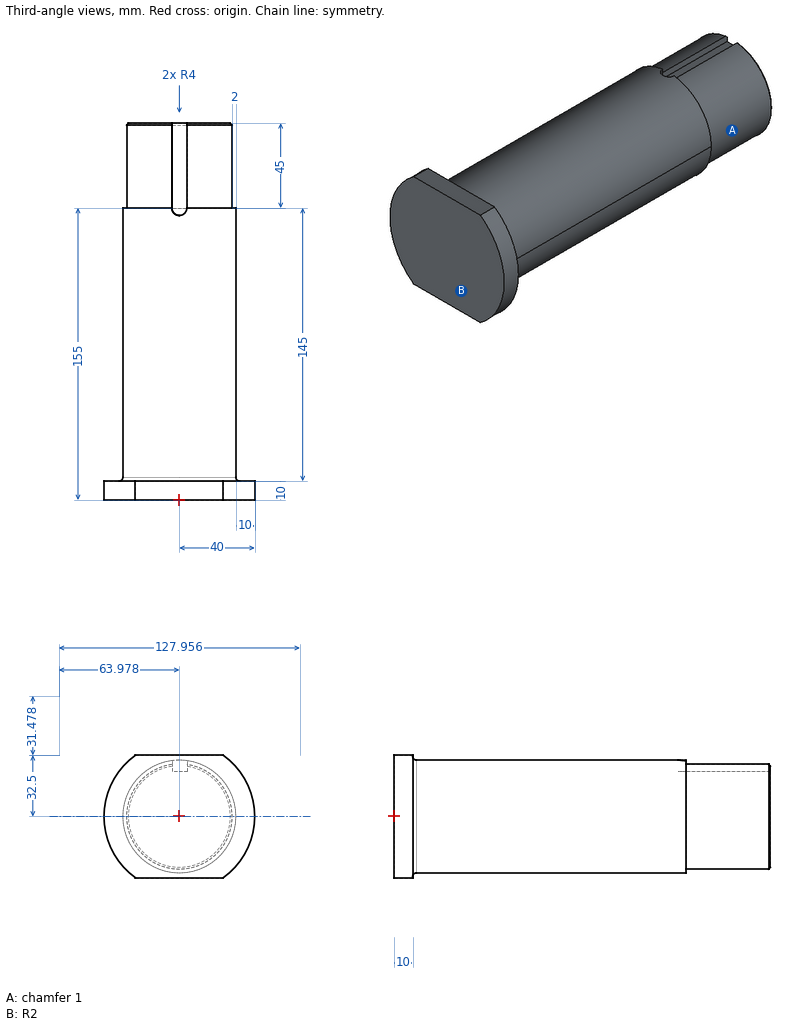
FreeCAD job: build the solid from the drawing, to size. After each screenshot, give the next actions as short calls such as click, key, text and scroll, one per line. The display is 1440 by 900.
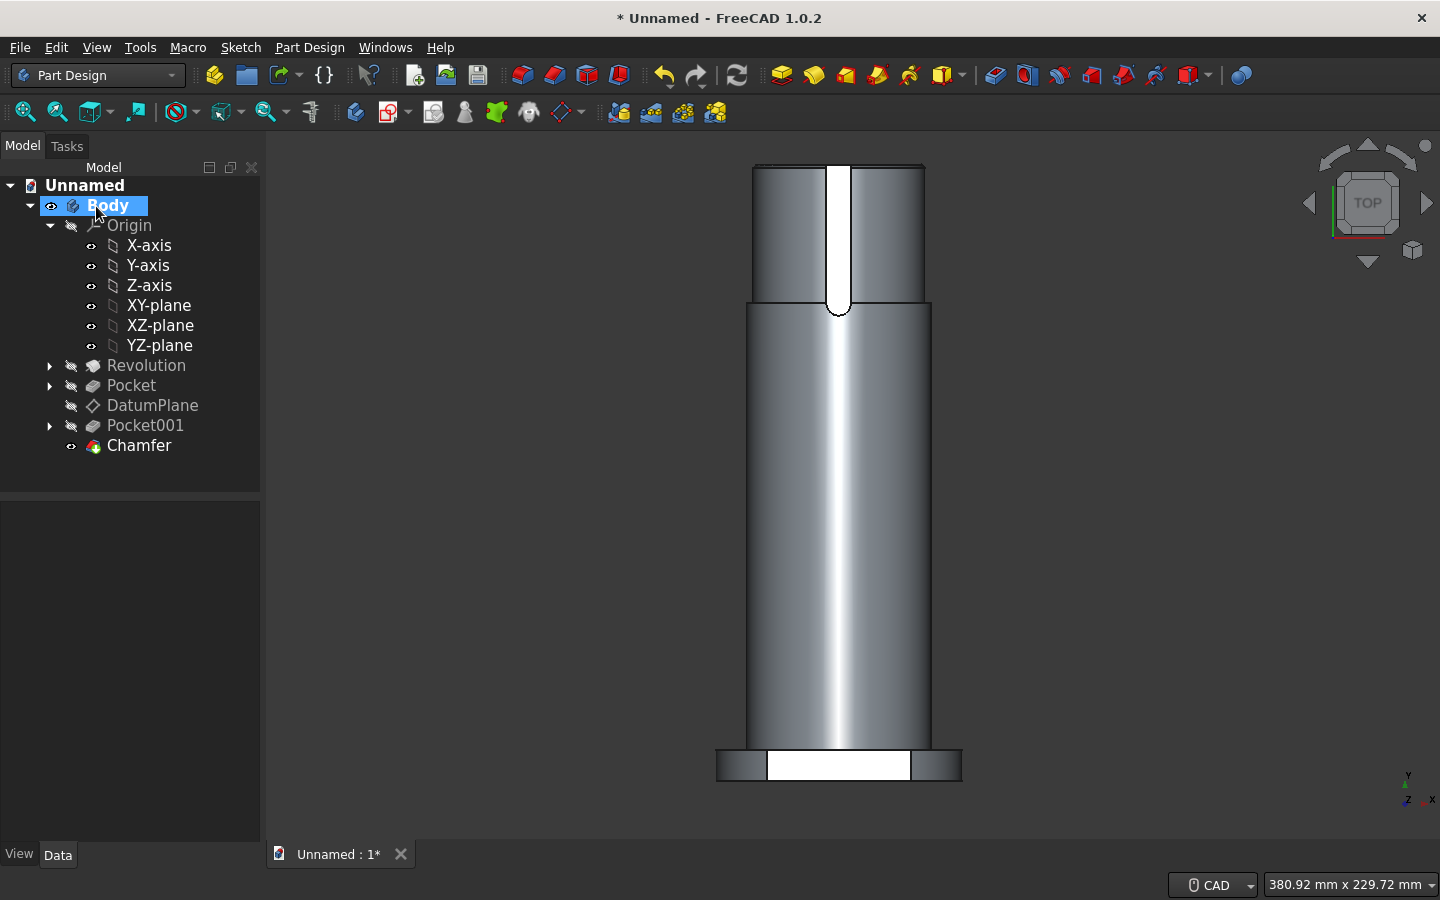
key(0)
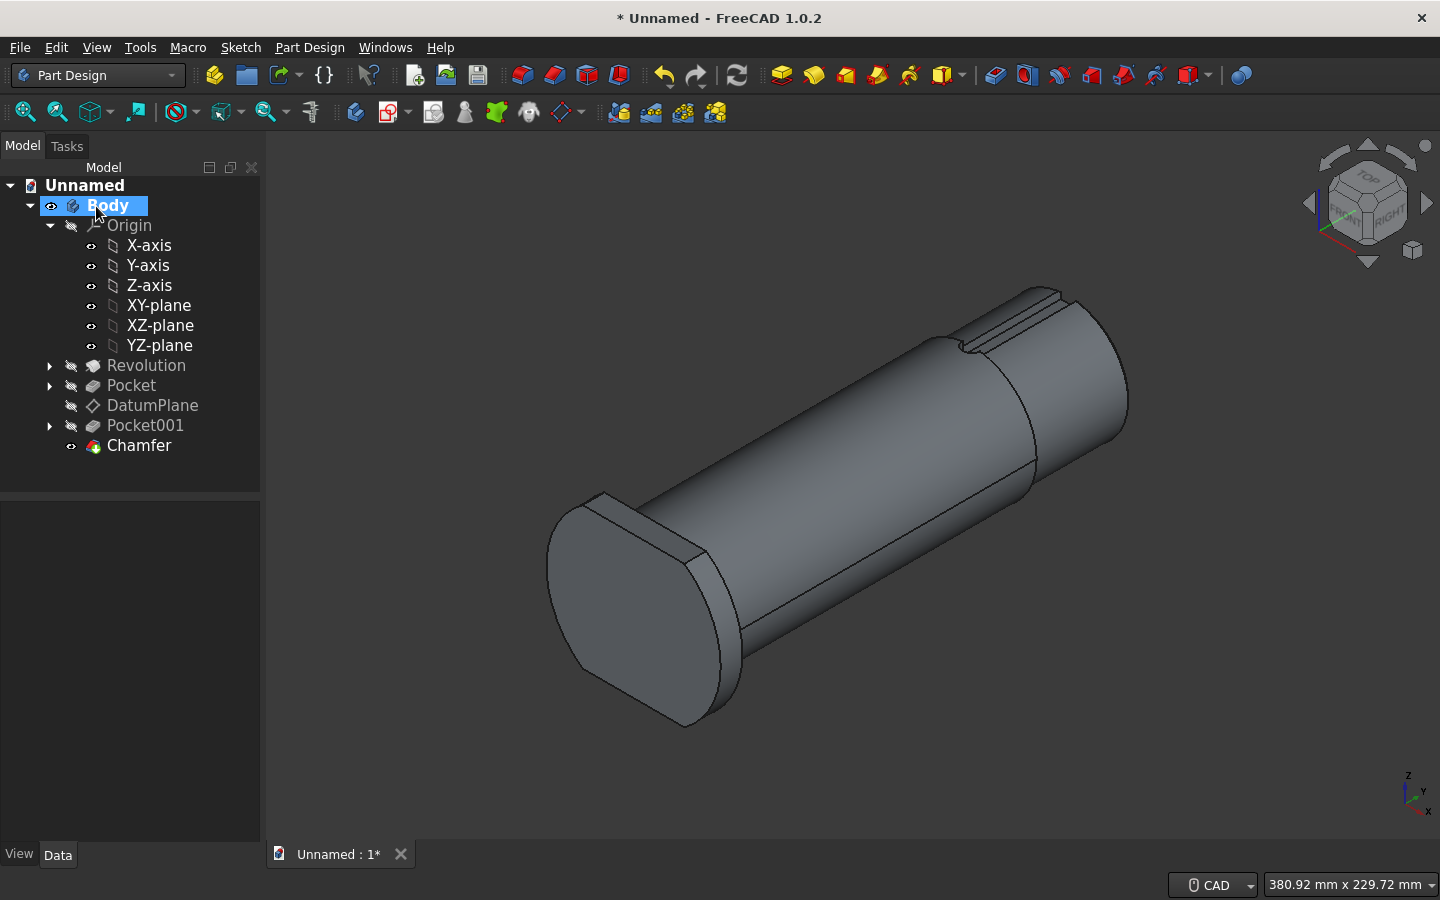
key(2)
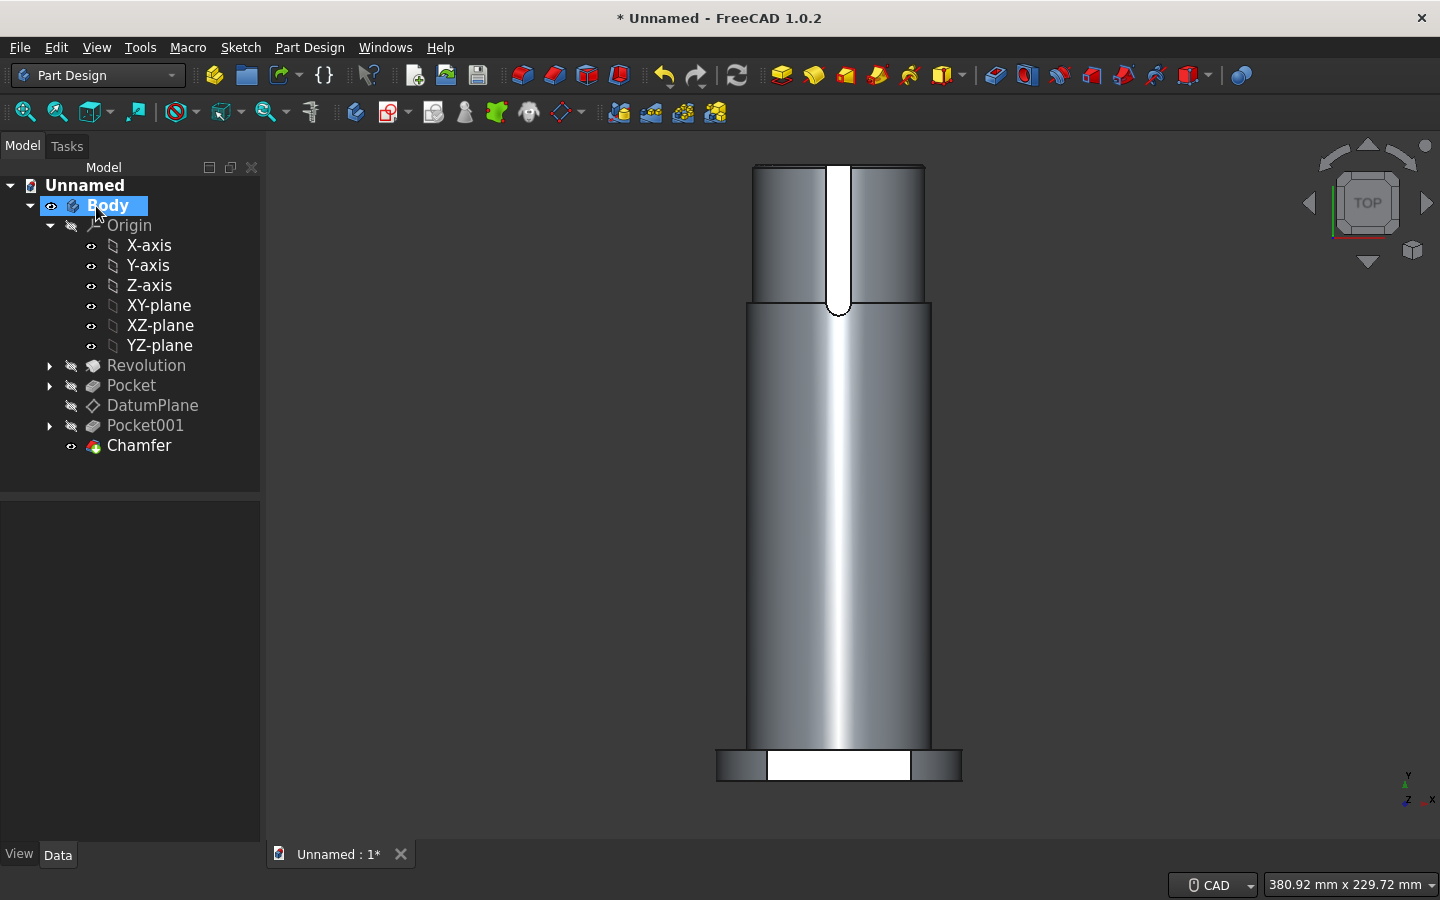
key(1)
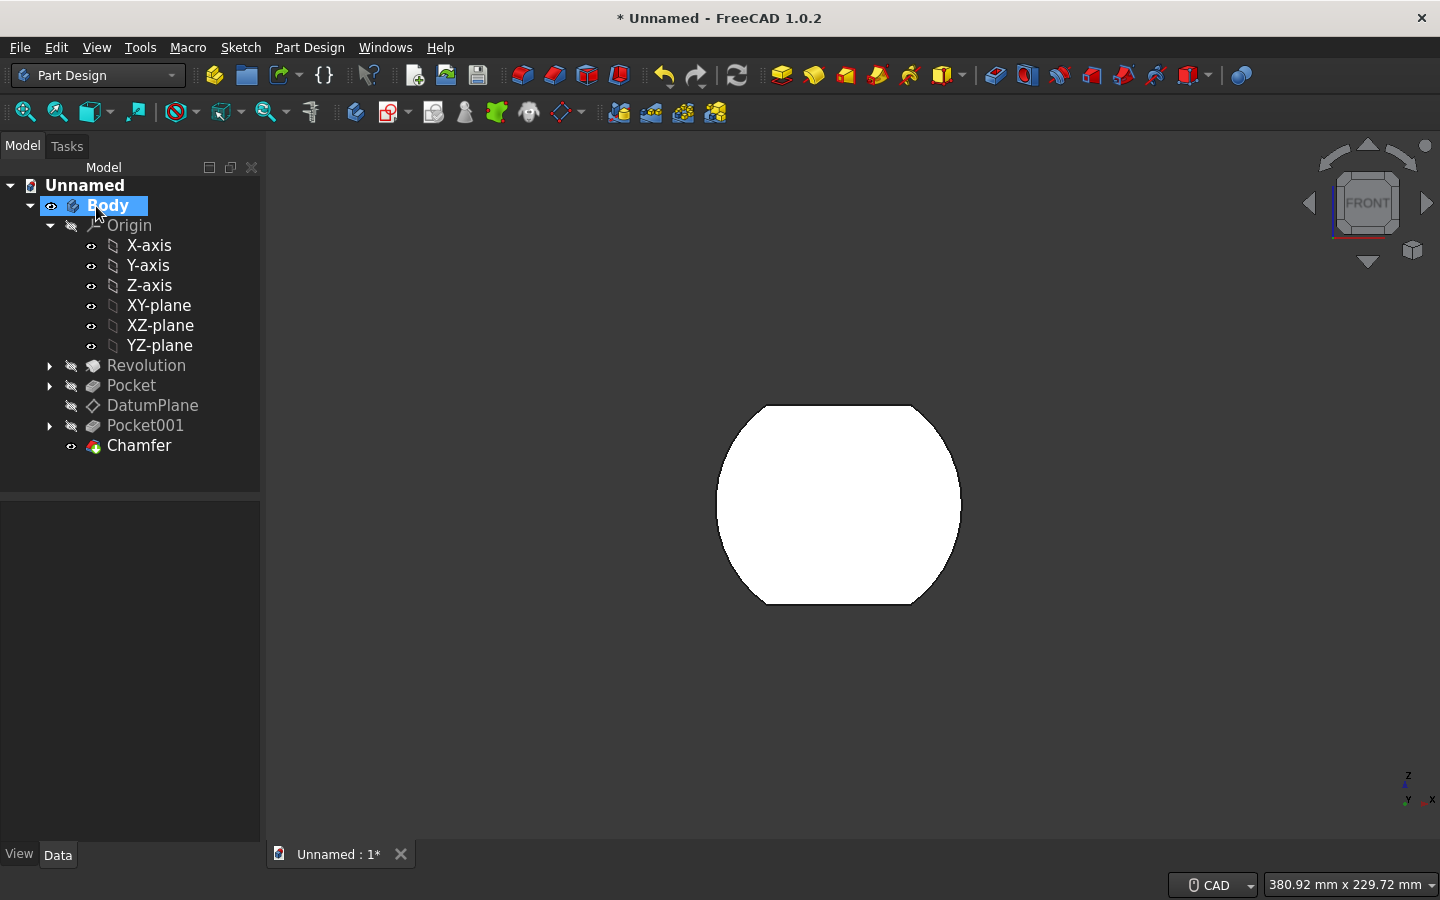
click(26, 112)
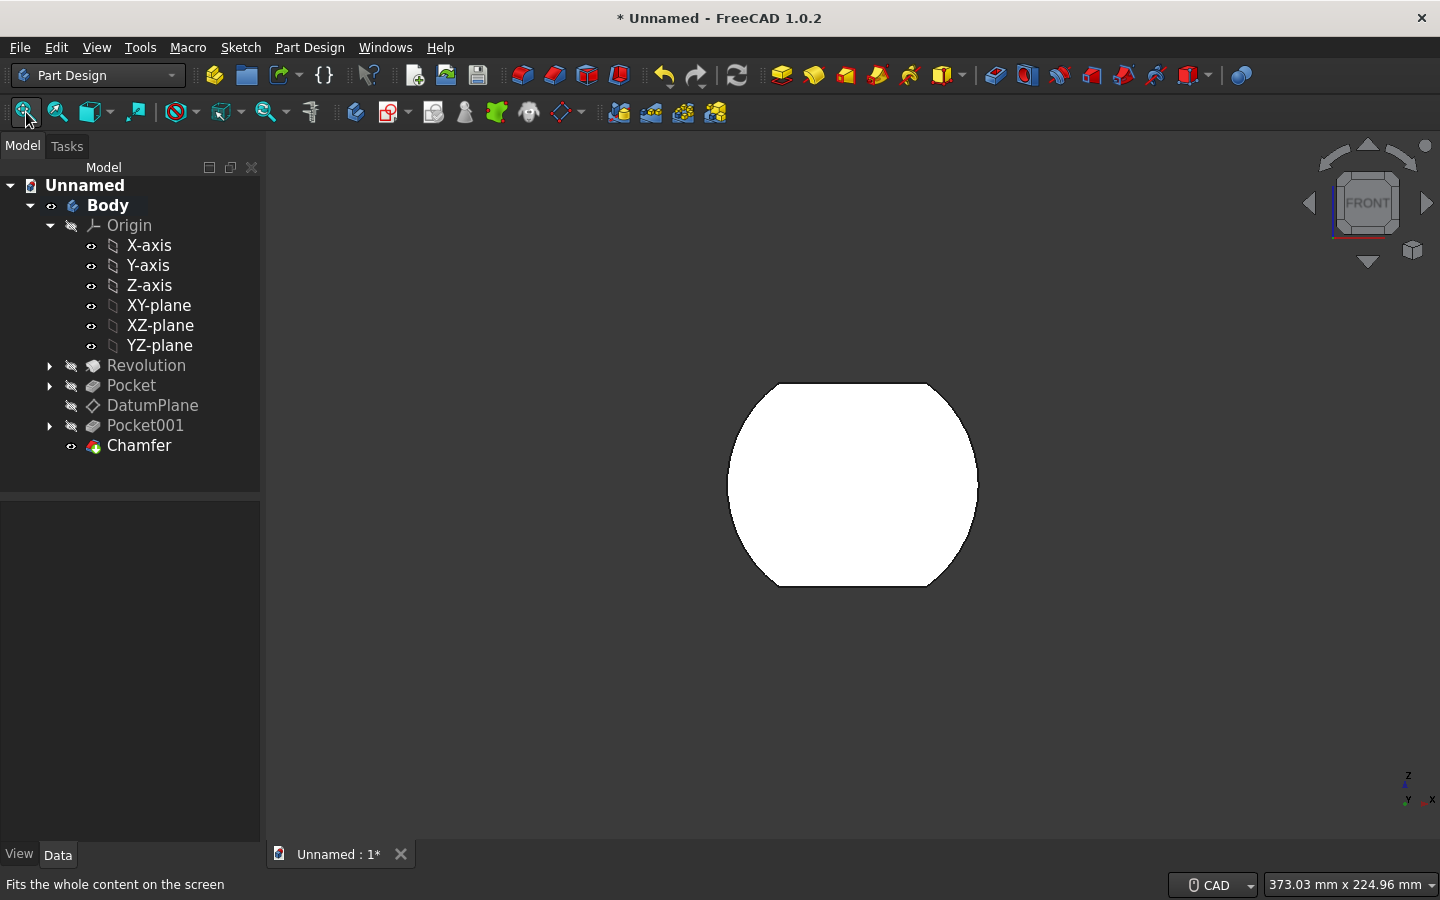
key(3)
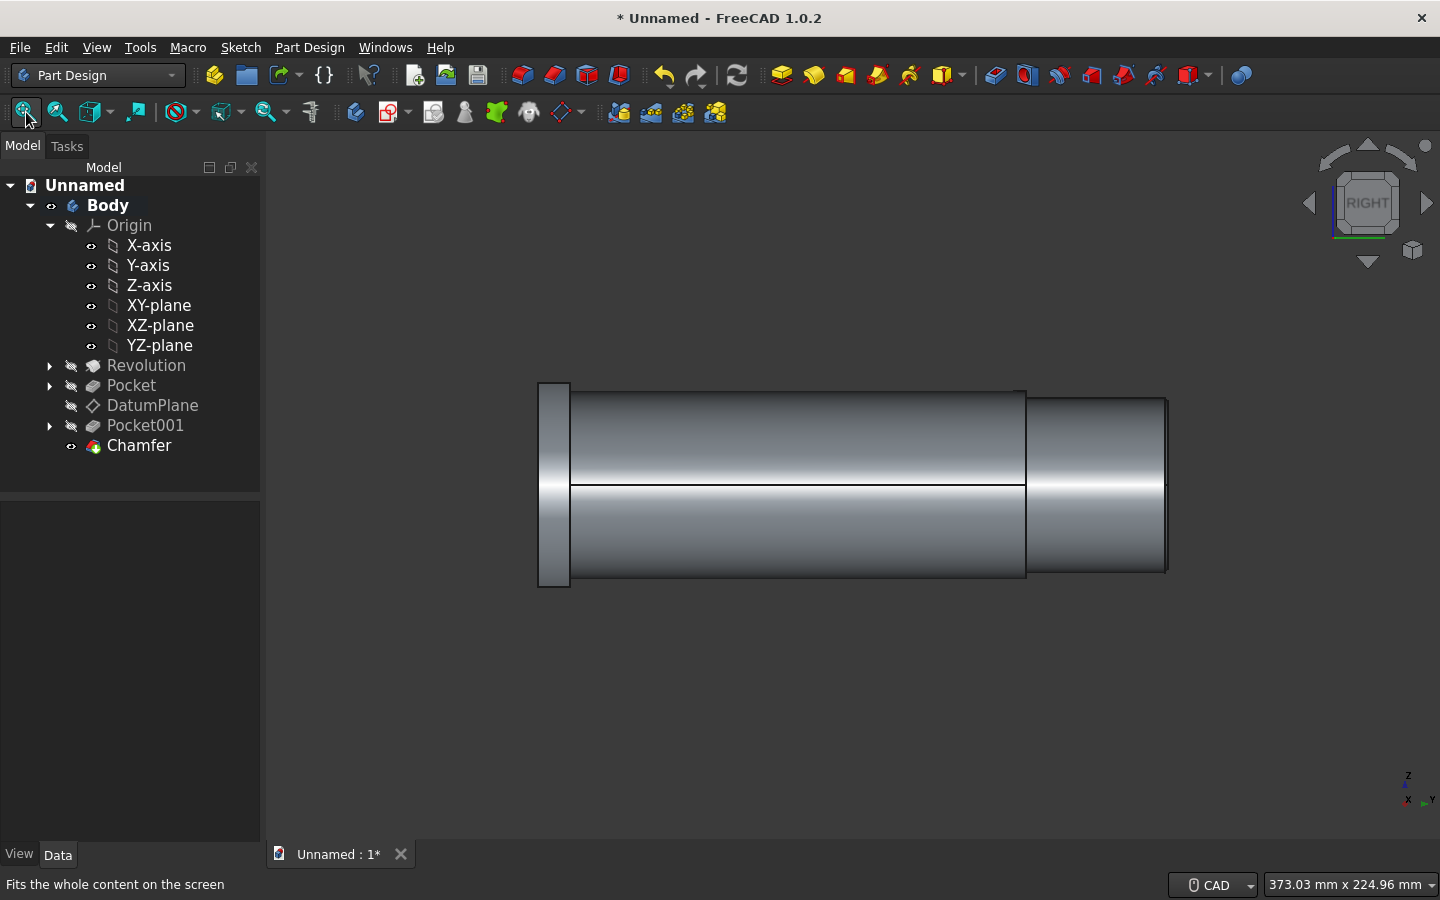
key(5)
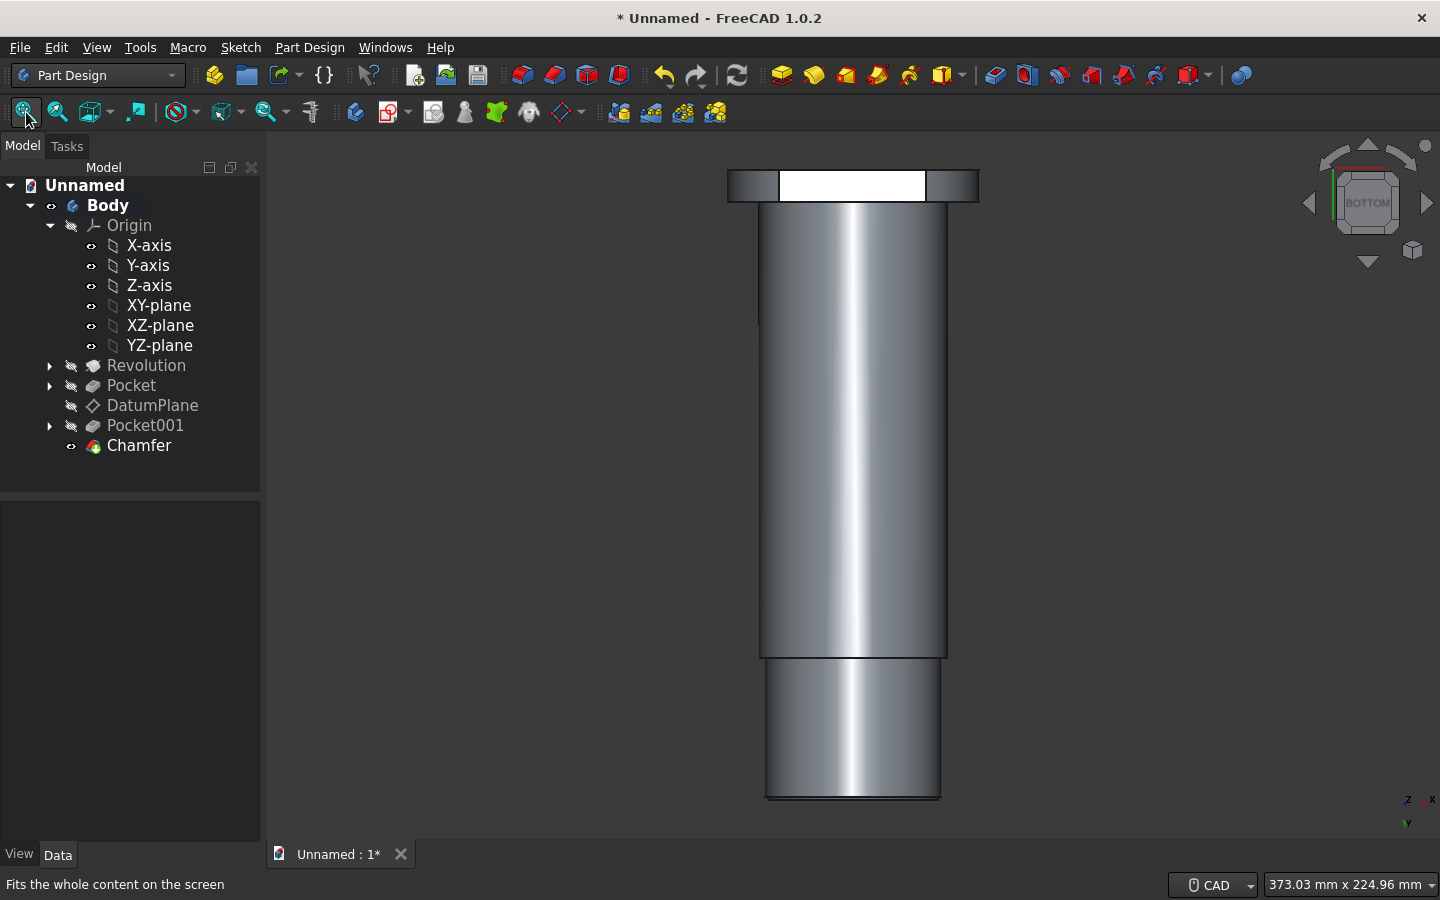
key(4)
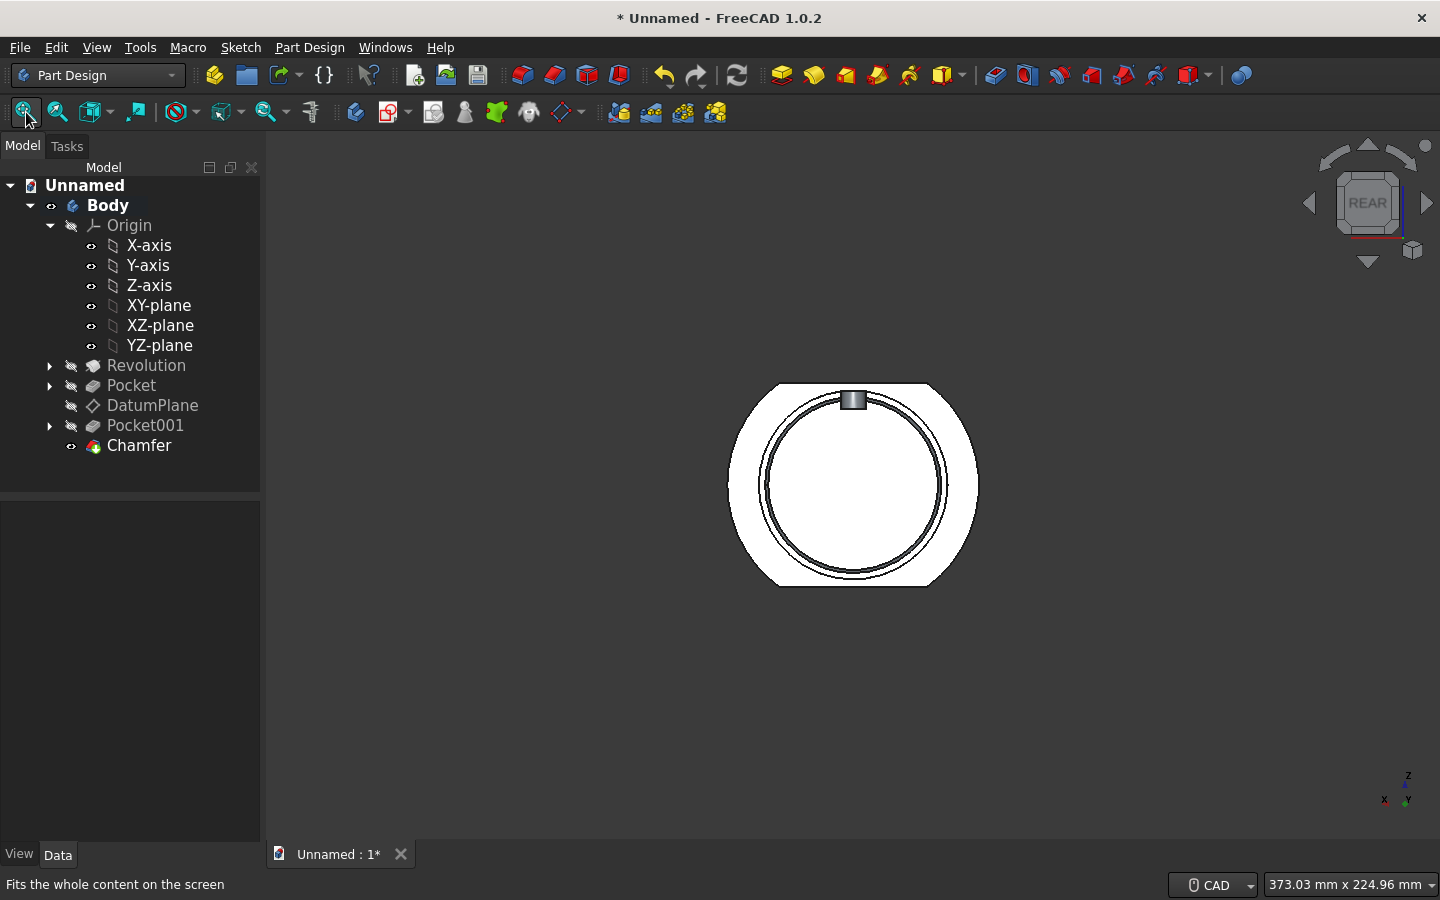
click(26, 112)